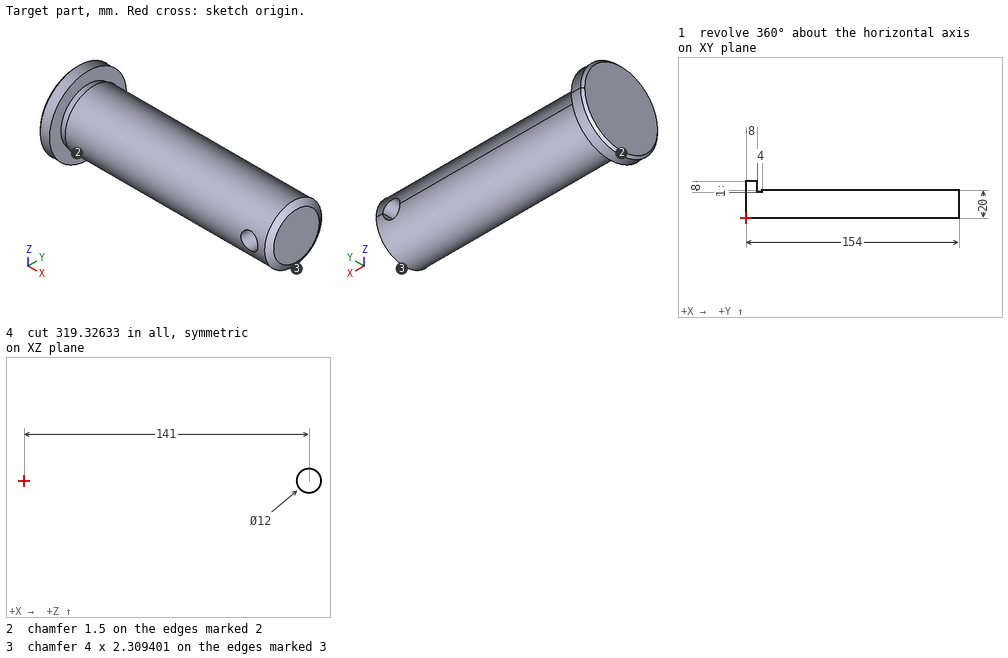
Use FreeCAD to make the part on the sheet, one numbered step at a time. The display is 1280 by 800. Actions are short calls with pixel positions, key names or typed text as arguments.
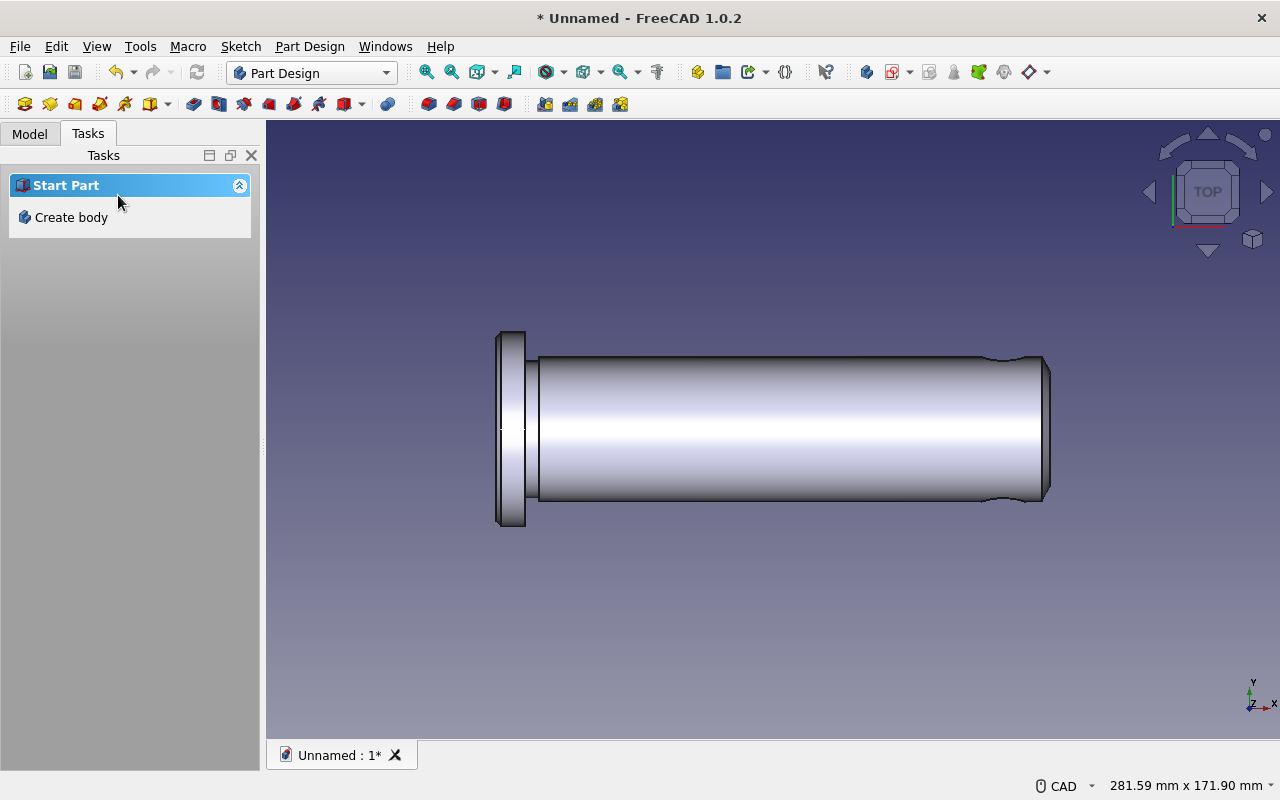
key(0)